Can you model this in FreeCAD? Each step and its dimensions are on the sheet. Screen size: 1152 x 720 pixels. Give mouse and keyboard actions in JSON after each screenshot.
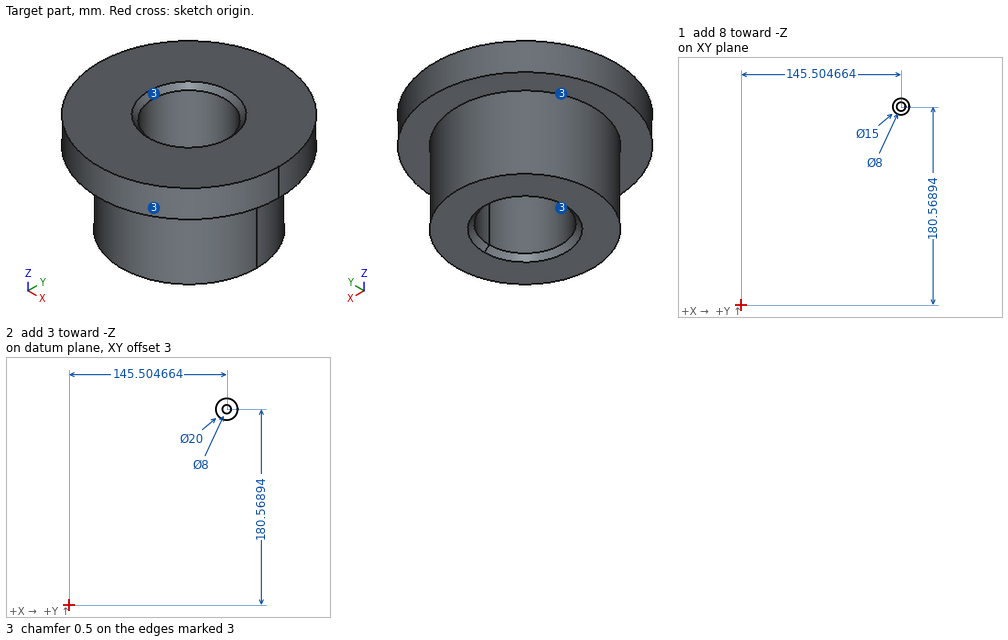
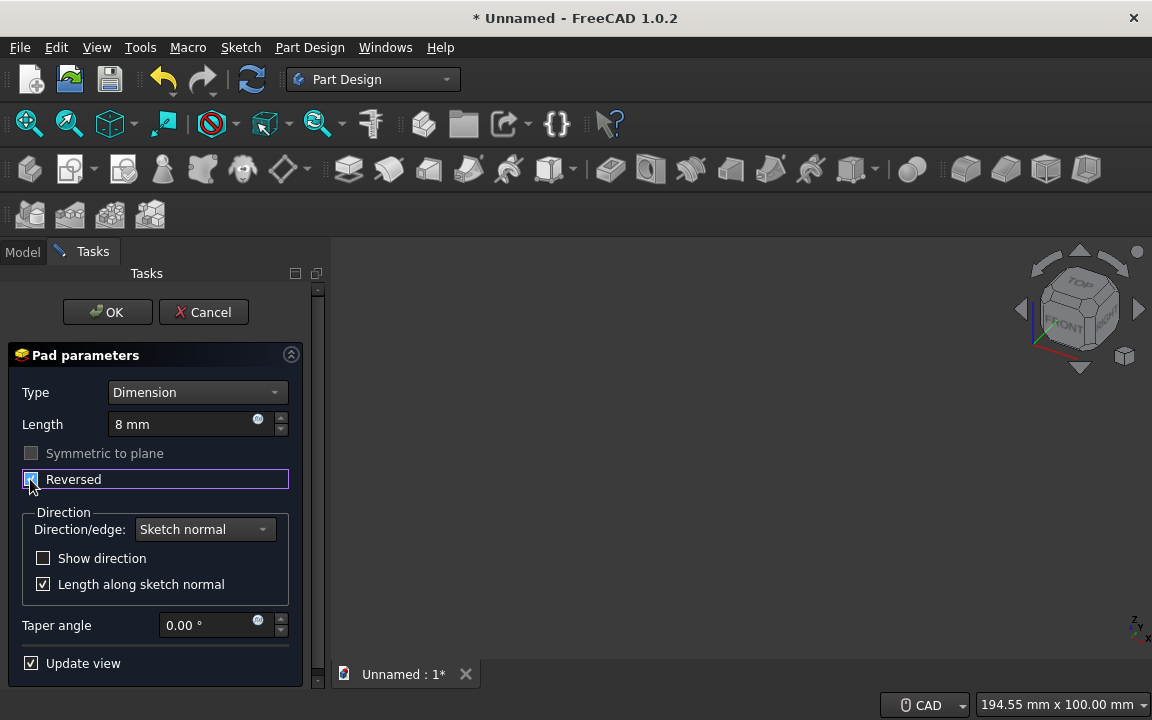
{"action": "left_click", "coordinate": [108, 312]}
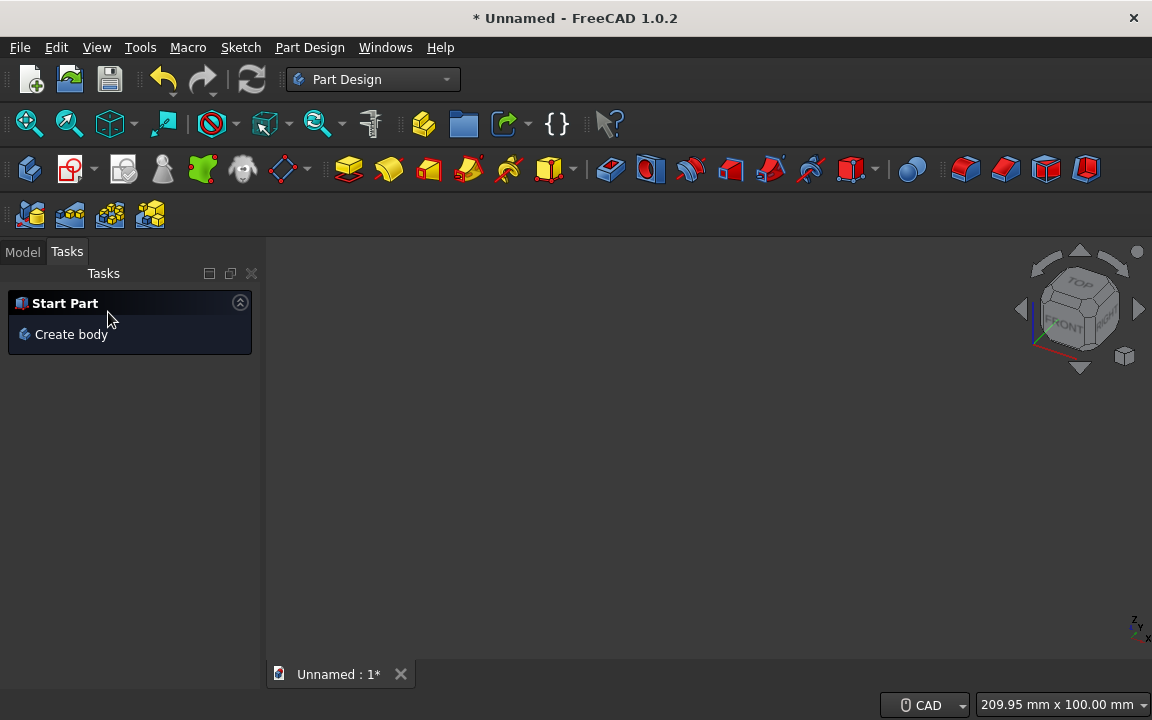
{"action": "key", "text": "v f"}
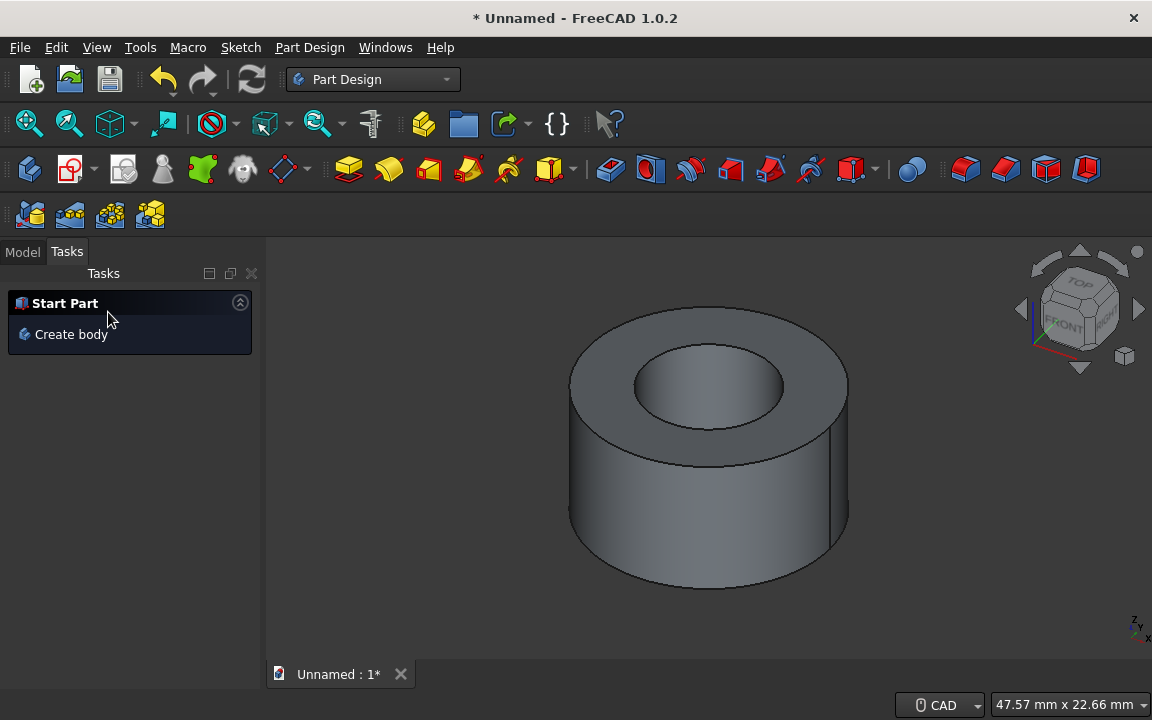
{"action": "left_click", "coordinate": [23, 251]}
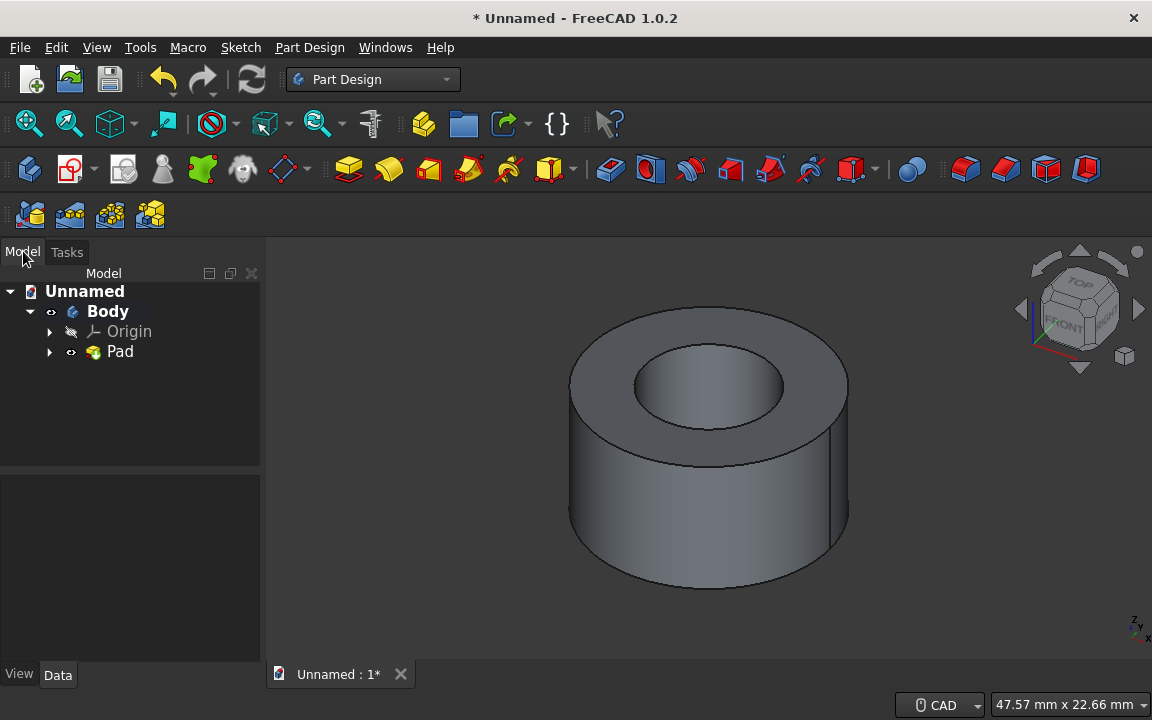
{"action": "left_click", "coordinate": [50, 332]}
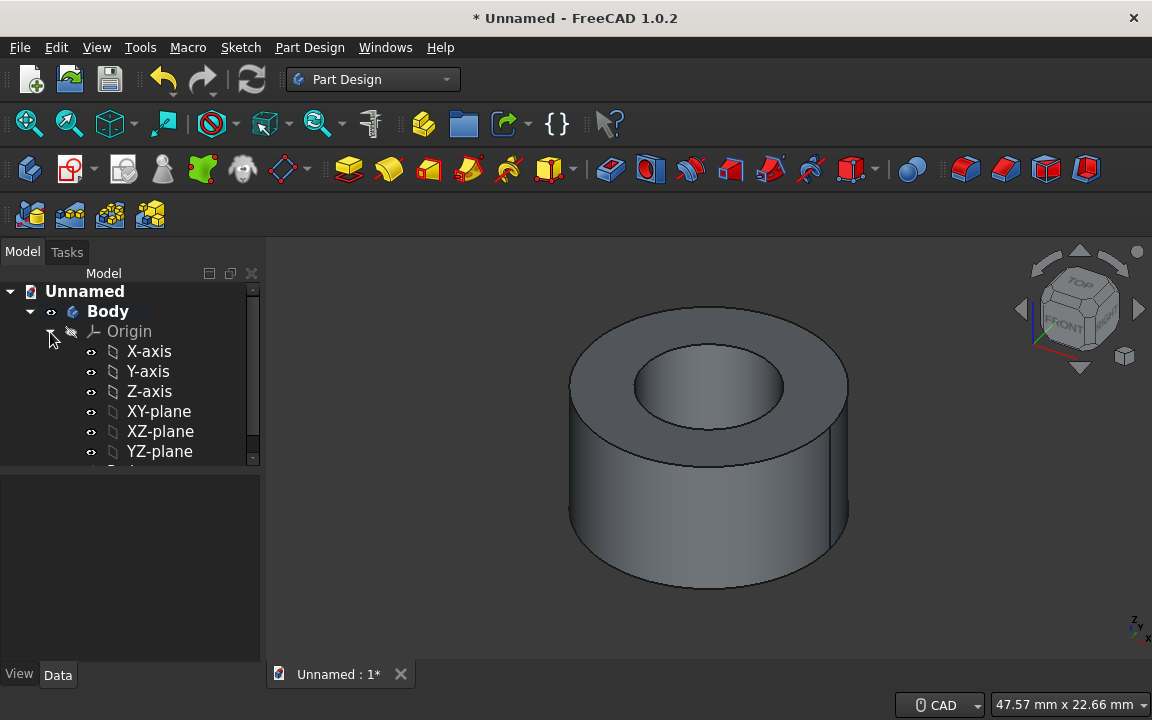
{"action": "left_click", "coordinate": [136, 412]}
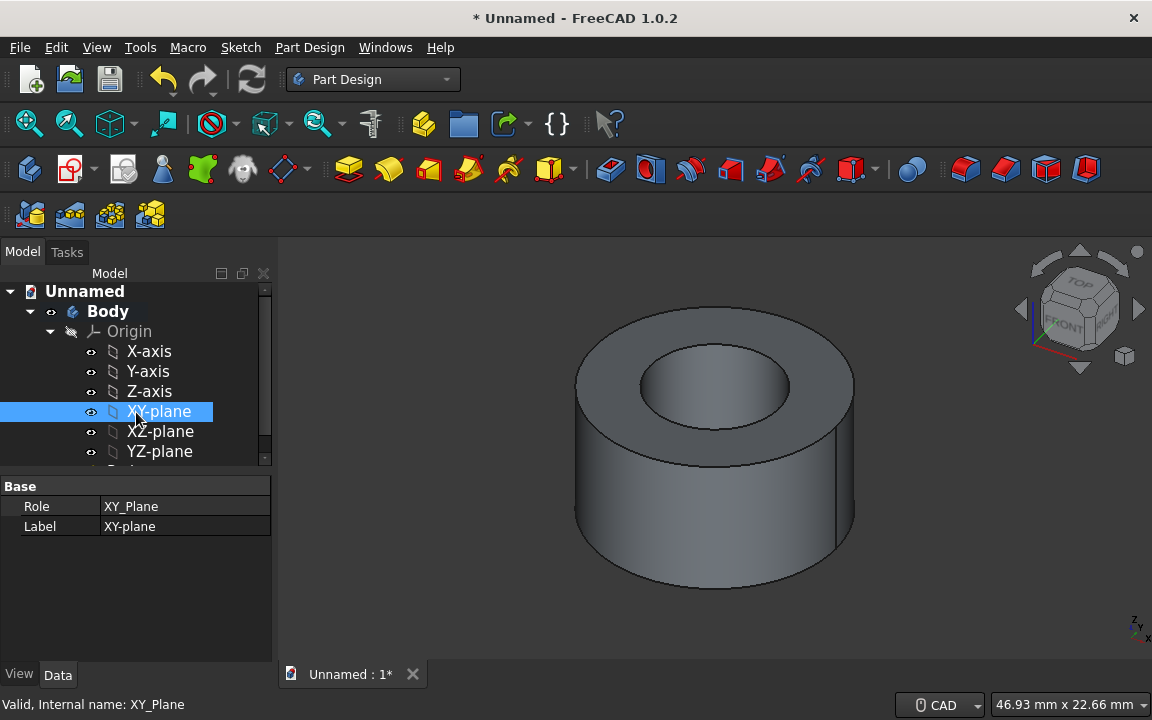
{"action": "left_click", "coordinate": [284, 170]}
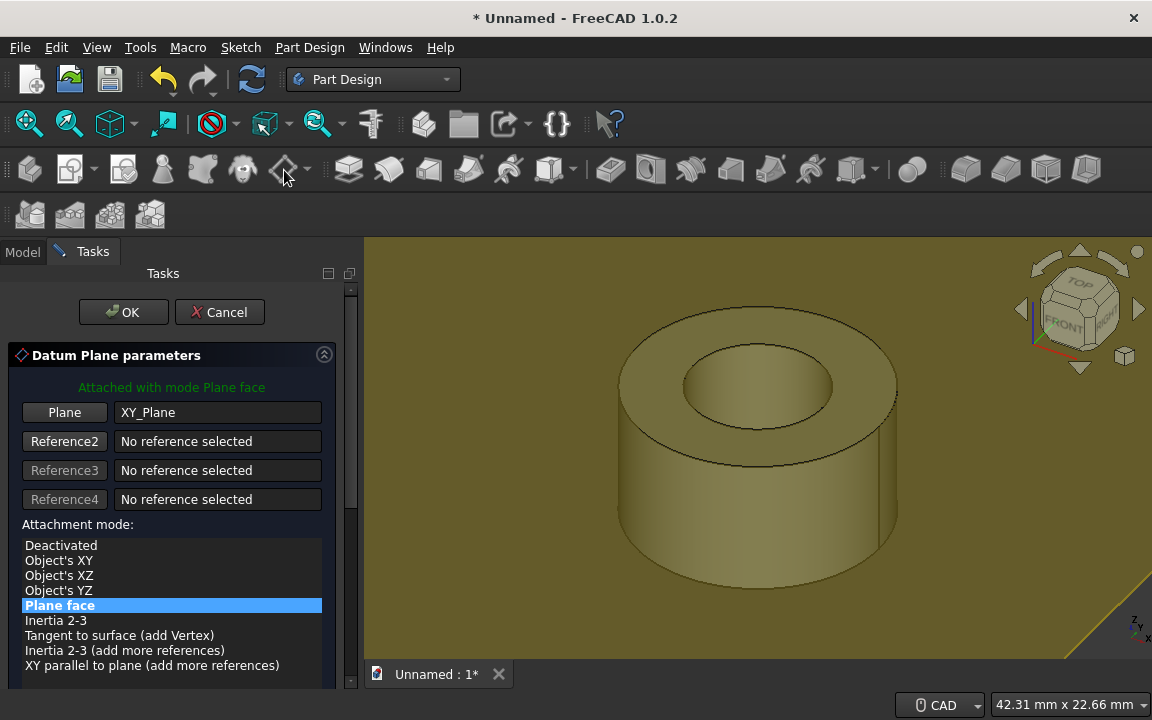
{"action": "scroll", "coordinate": [351, 486], "scroll_direction": "down", "scroll_amount": 4}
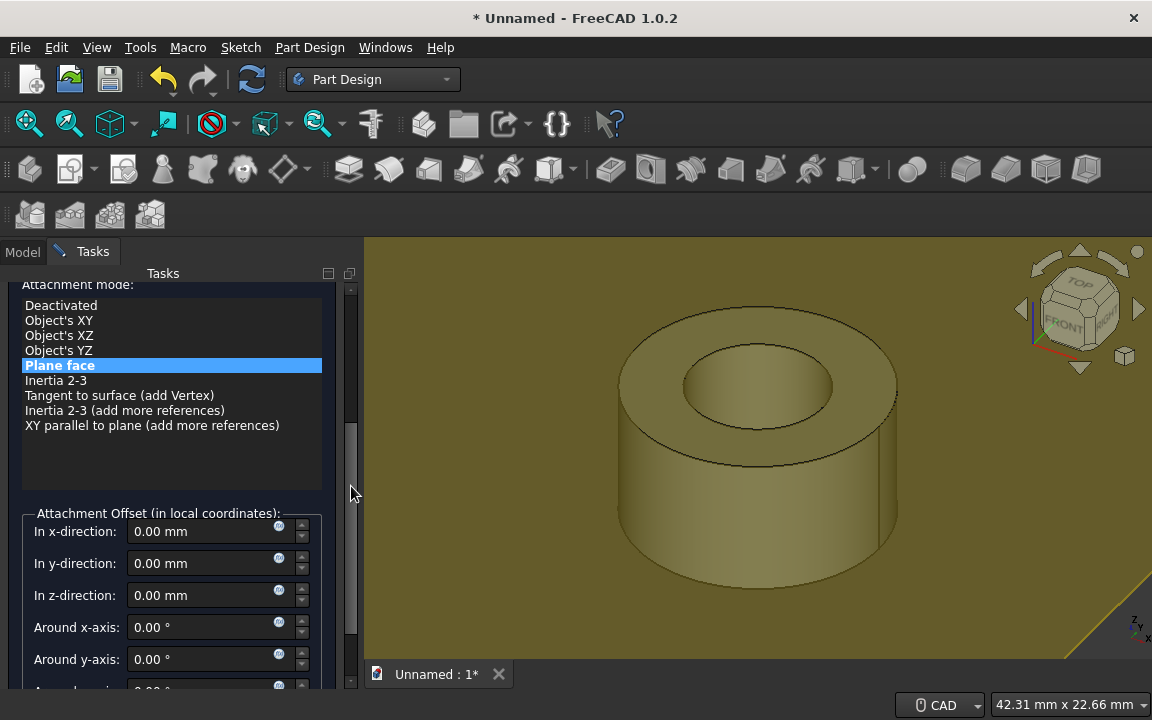
{"action": "triple_click", "coordinate": [210, 595]}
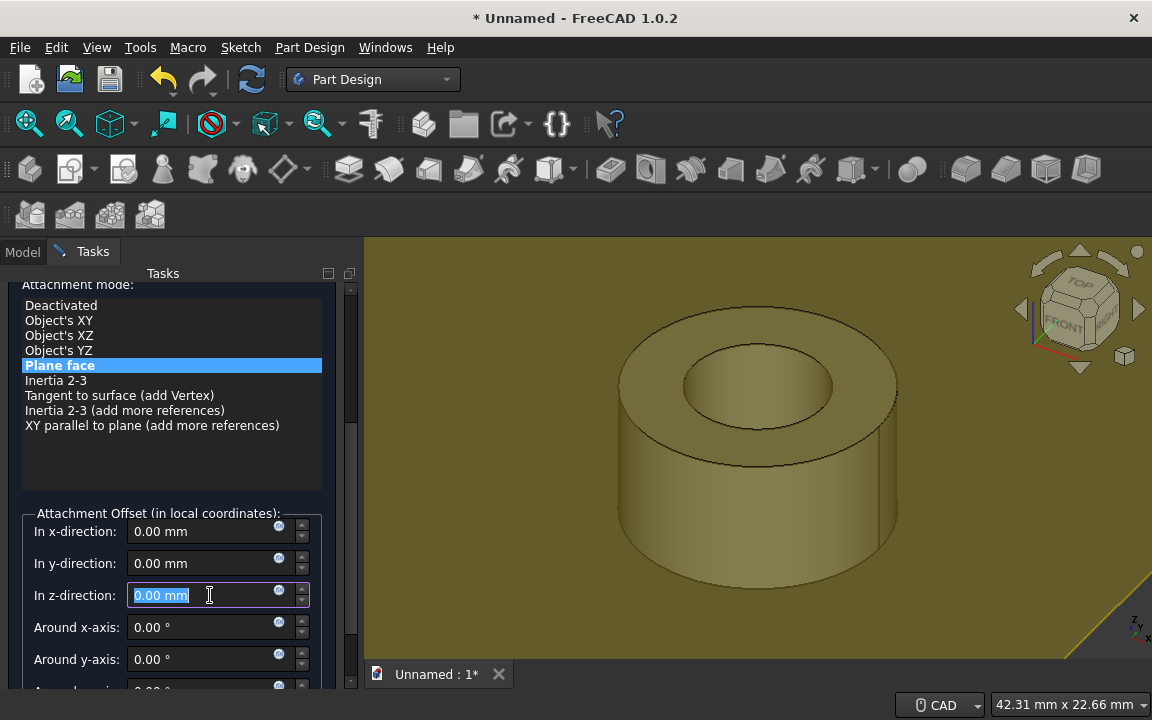
{"action": "type", "text": "3"}
{"action": "key", "text": "Tab"}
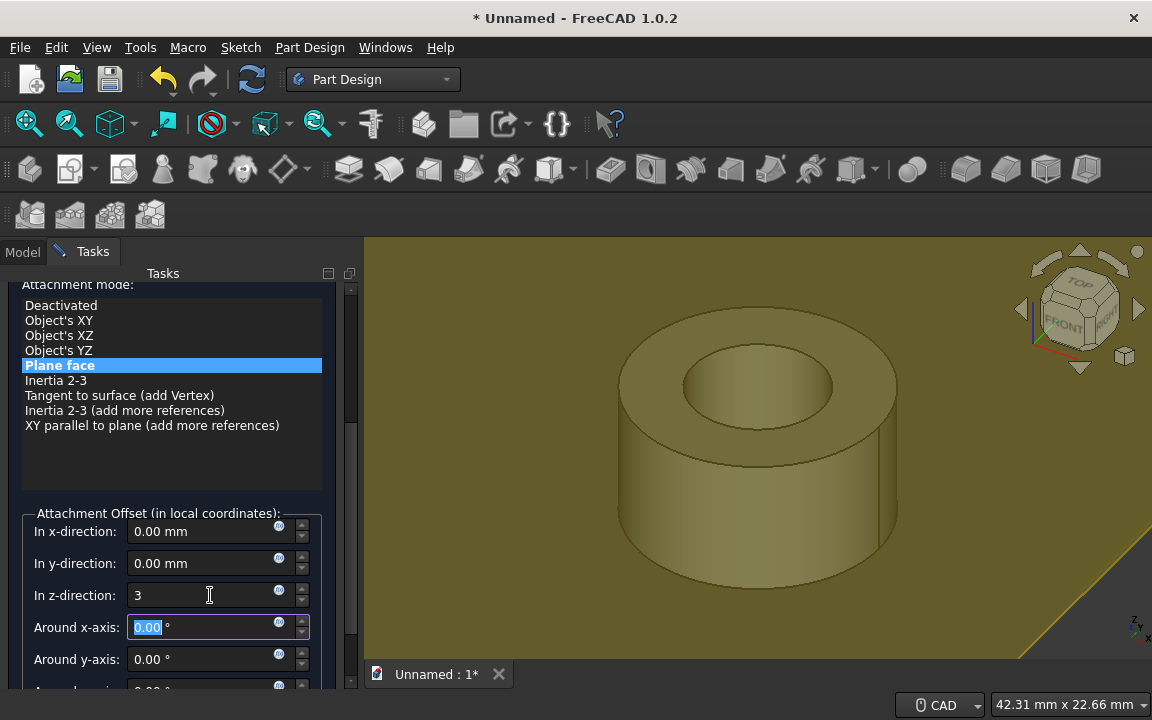
{"action": "scroll", "coordinate": [351, 486], "scroll_direction": "up", "scroll_amount": 5}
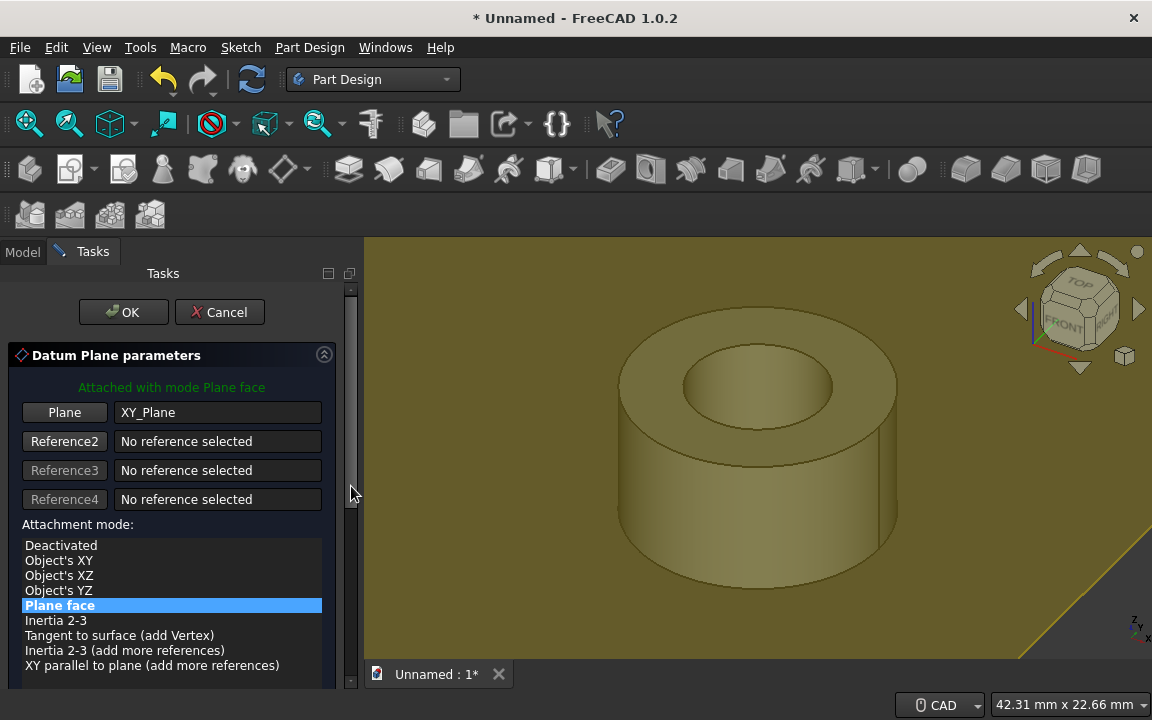
{"action": "left_click", "coordinate": [124, 312]}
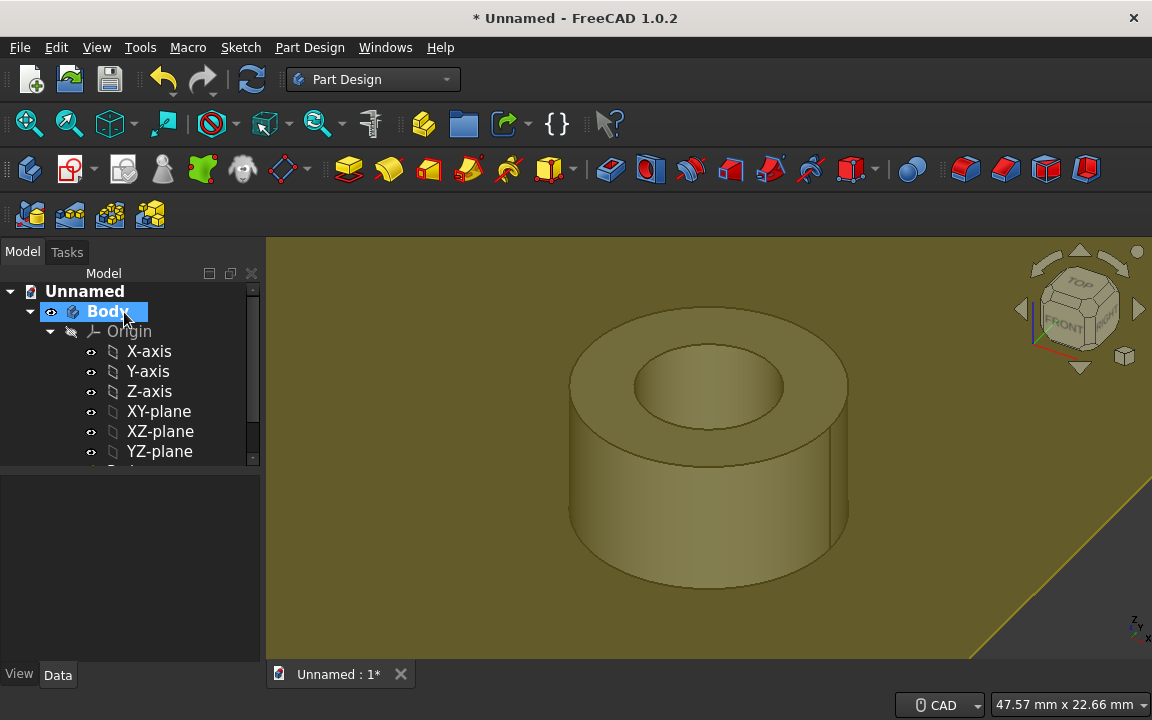
{"action": "scroll", "coordinate": [100, 367], "scroll_direction": "down", "scroll_amount": 3}